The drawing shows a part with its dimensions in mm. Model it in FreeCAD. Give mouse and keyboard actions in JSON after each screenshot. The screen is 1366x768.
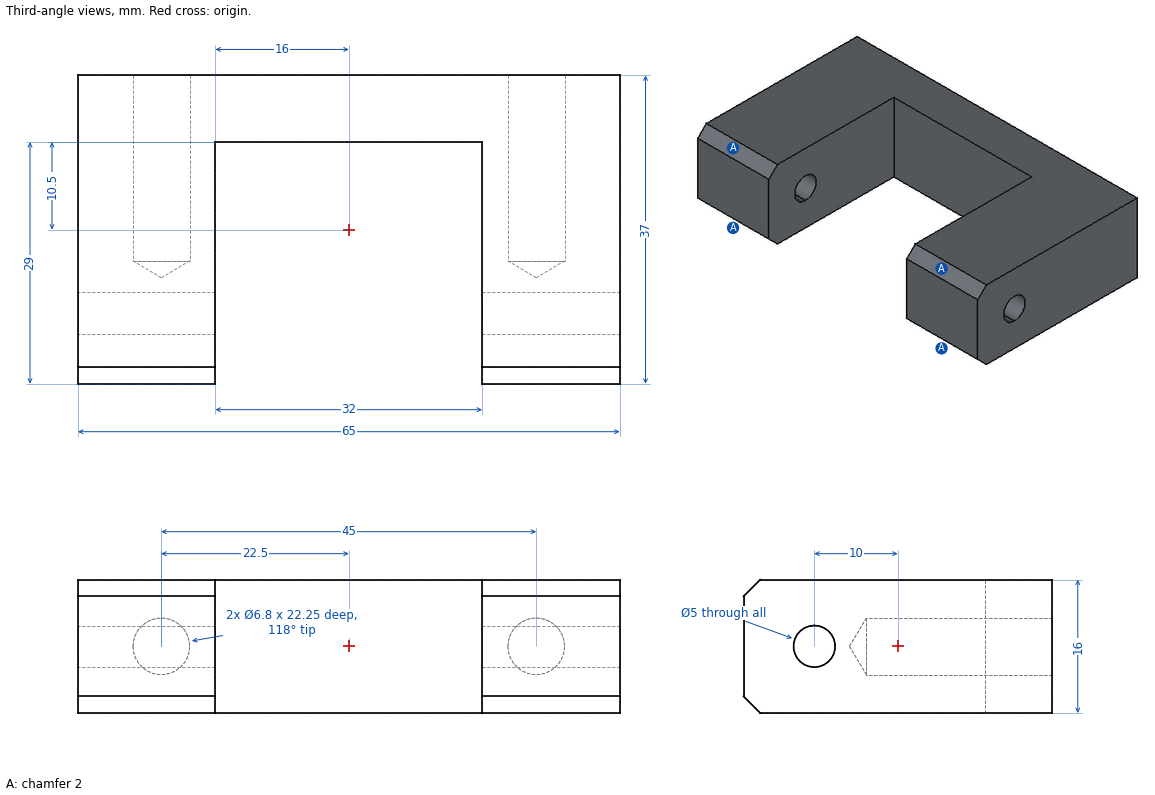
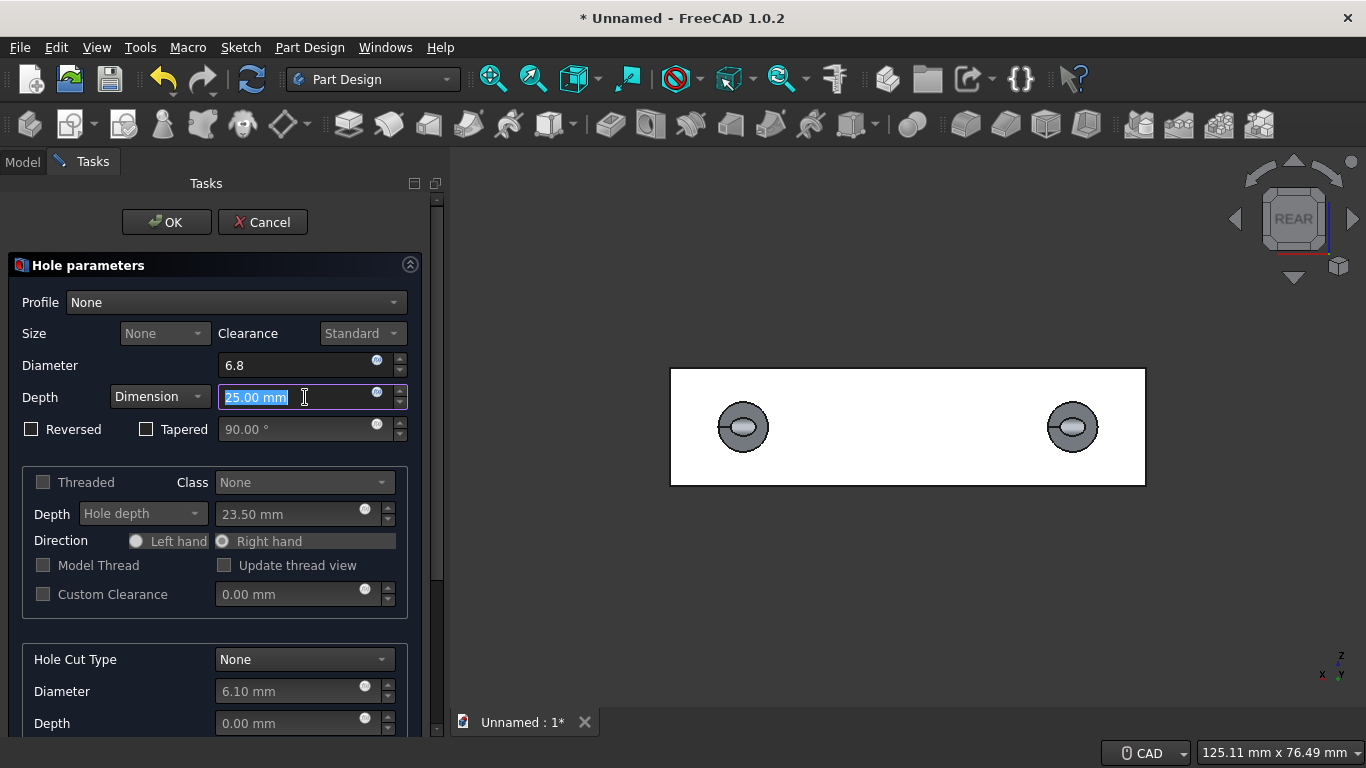
{"action": "type", "text": "22.25"}
{"action": "key", "text": "Tab"}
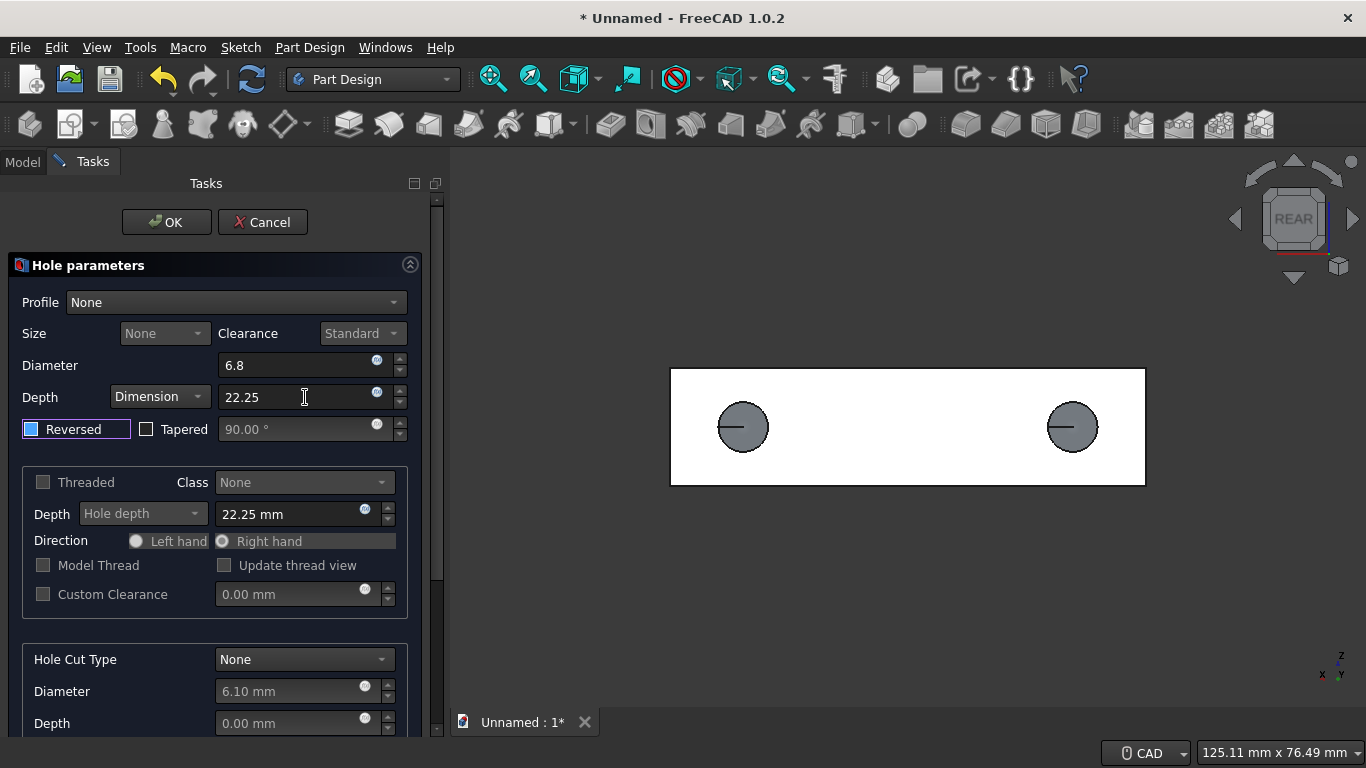
{"action": "left_click", "coordinate": [167, 222]}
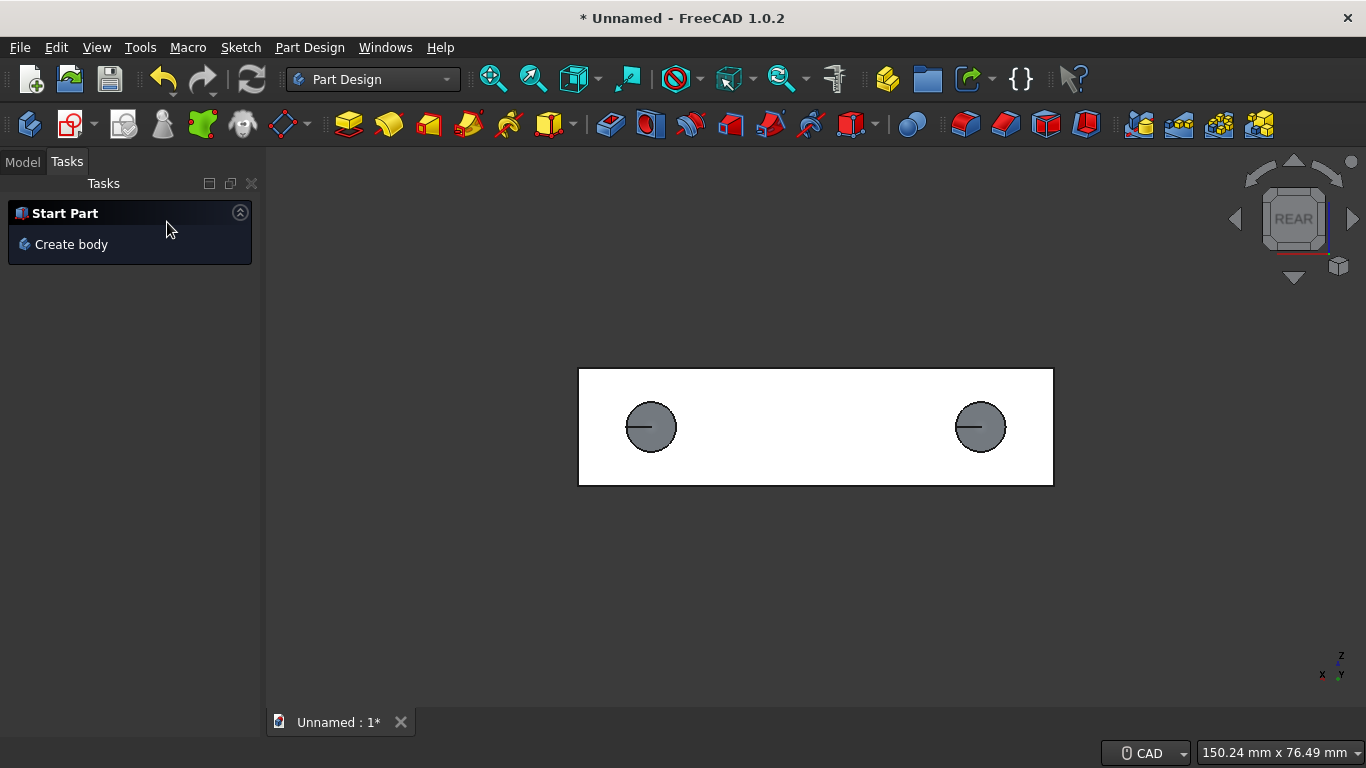
{"action": "left_click", "coordinate": [494, 80]}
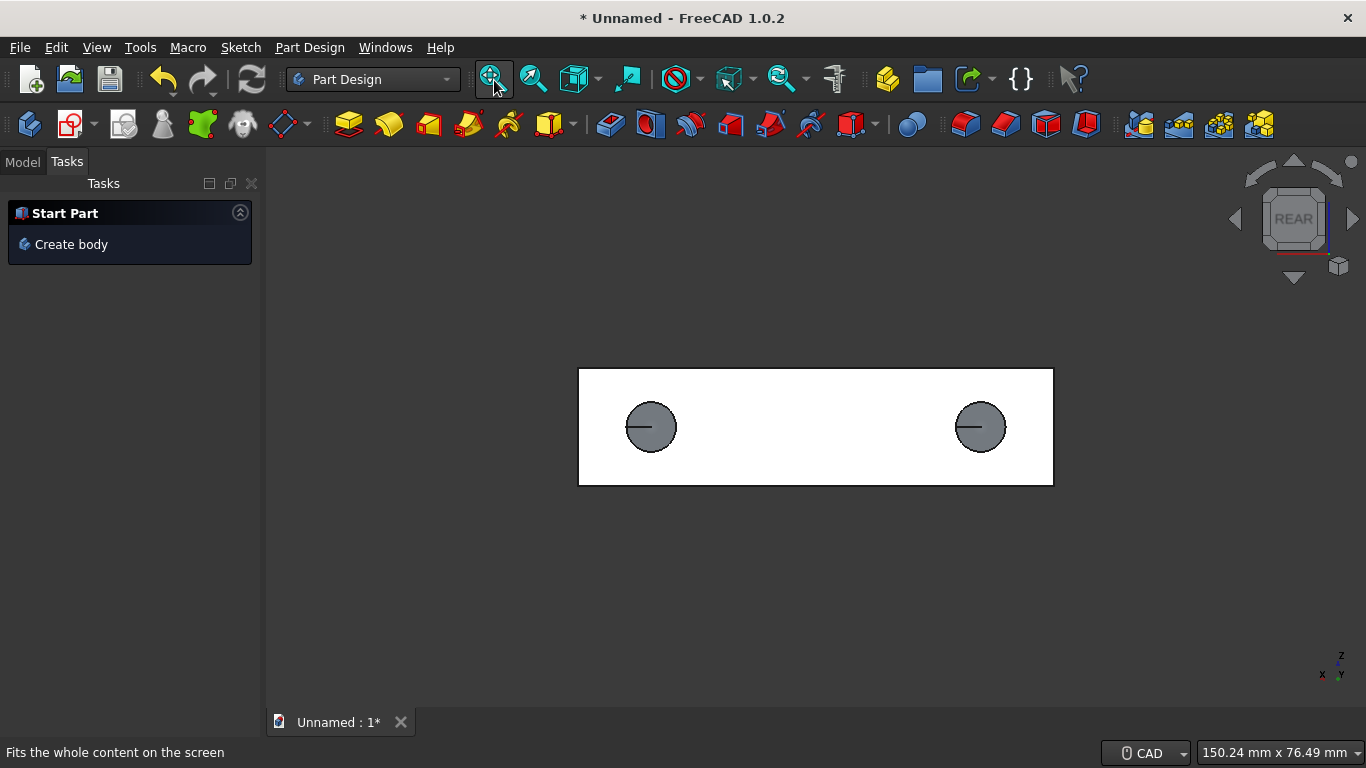
{"action": "key", "text": "0"}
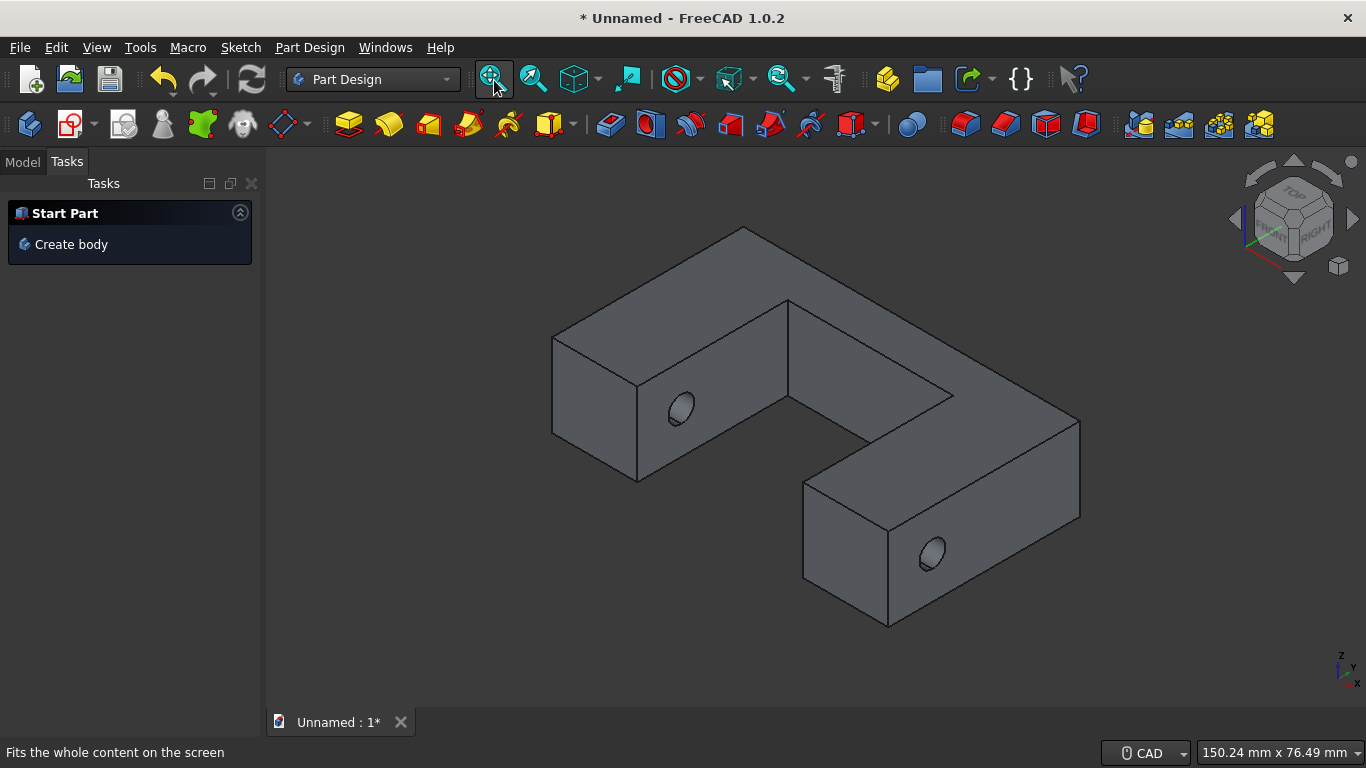
{"action": "left_click", "coordinate": [846, 506]}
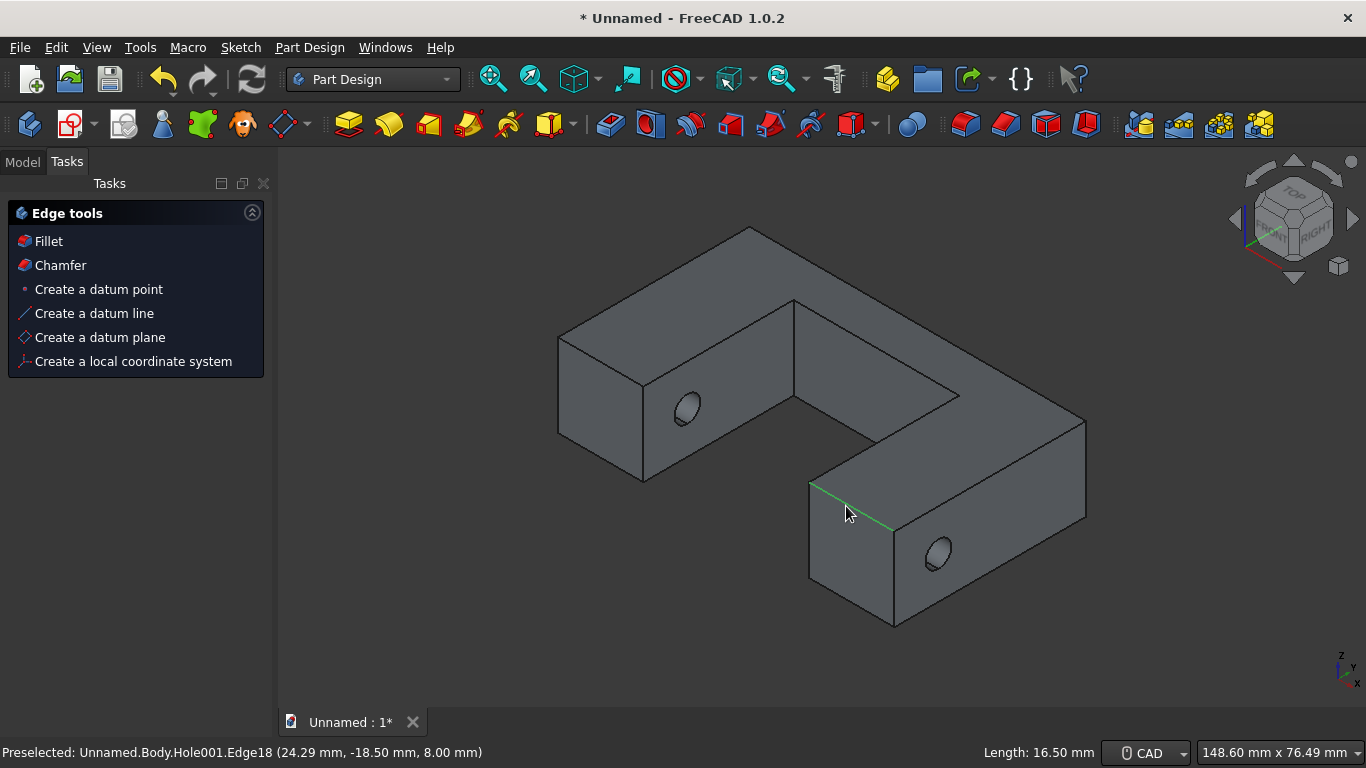
{"action": "left_click", "coordinate": [601, 361], "text": "ctrl"}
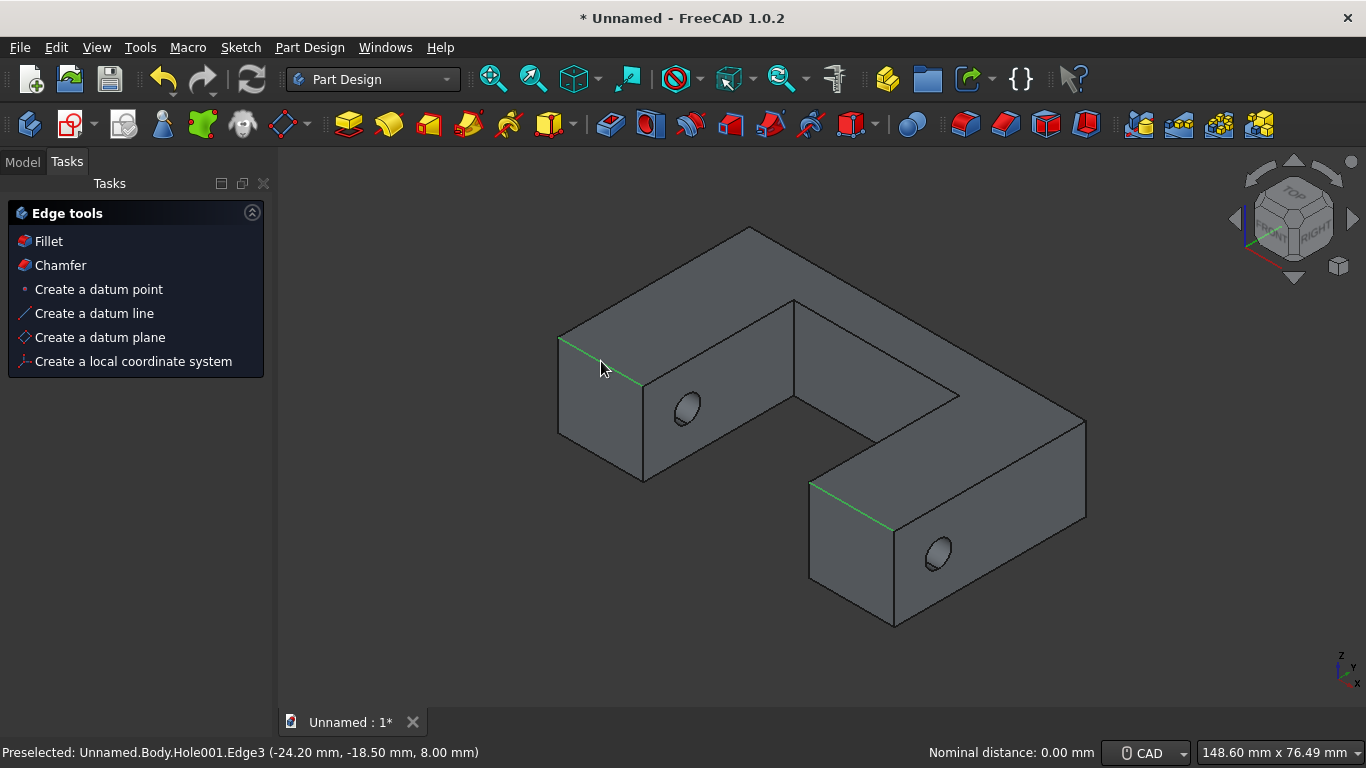
{"action": "key", "text": "2"}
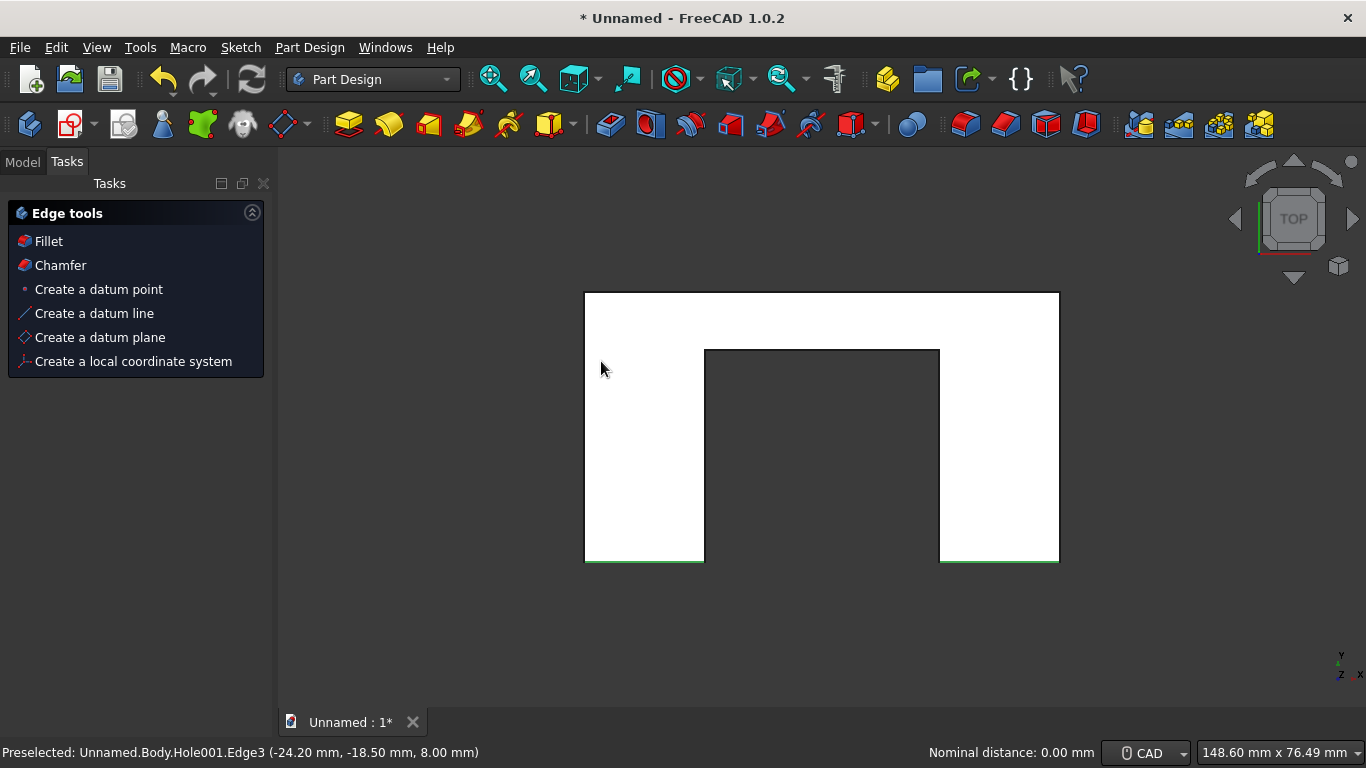
{"action": "key", "text": "1"}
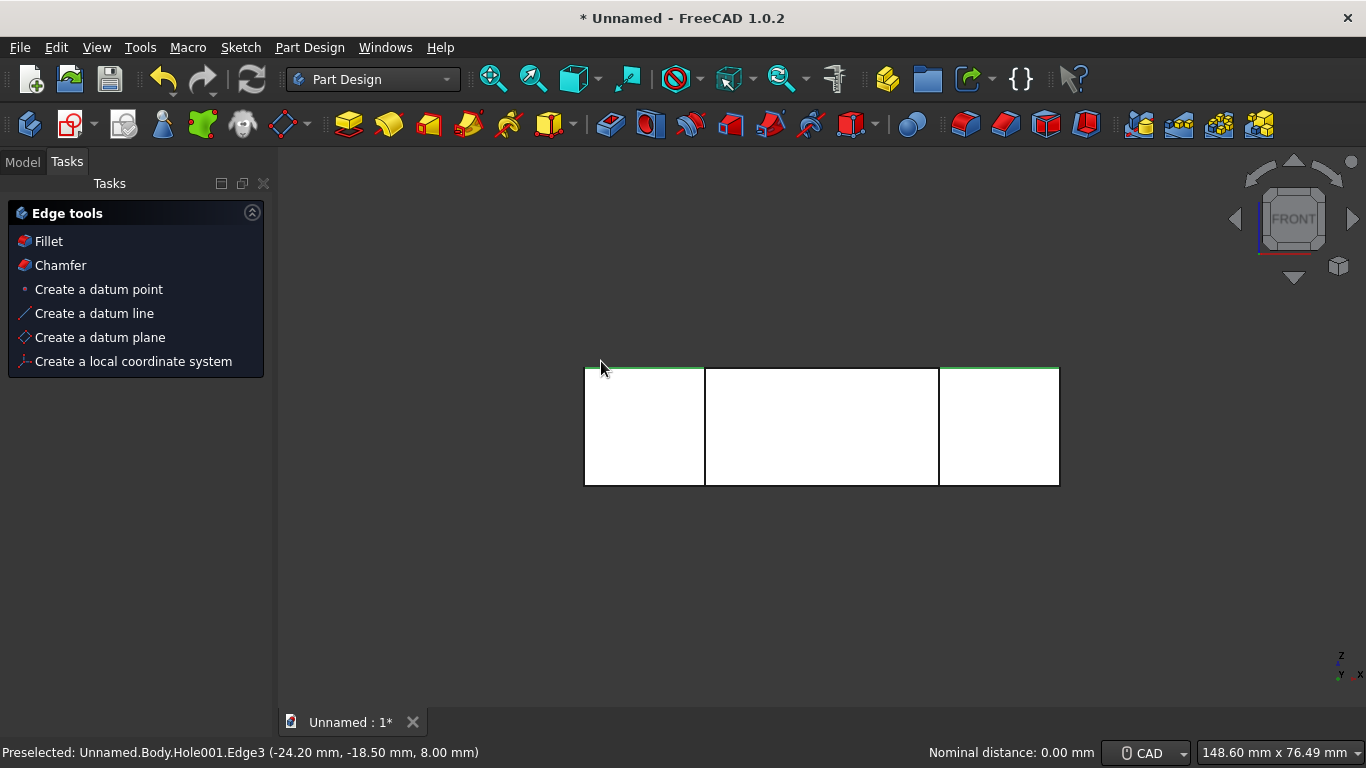
{"action": "left_click", "coordinate": [494, 80]}